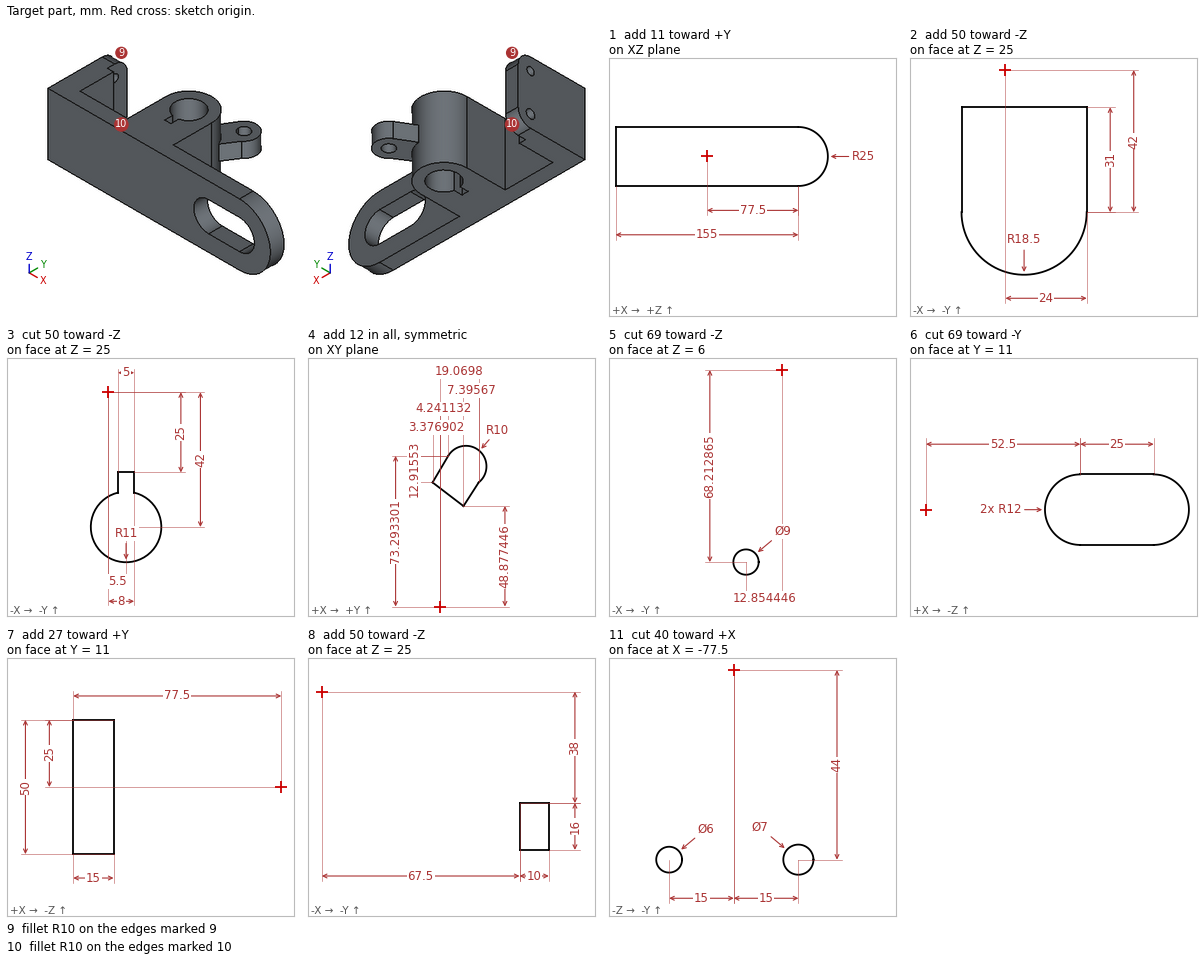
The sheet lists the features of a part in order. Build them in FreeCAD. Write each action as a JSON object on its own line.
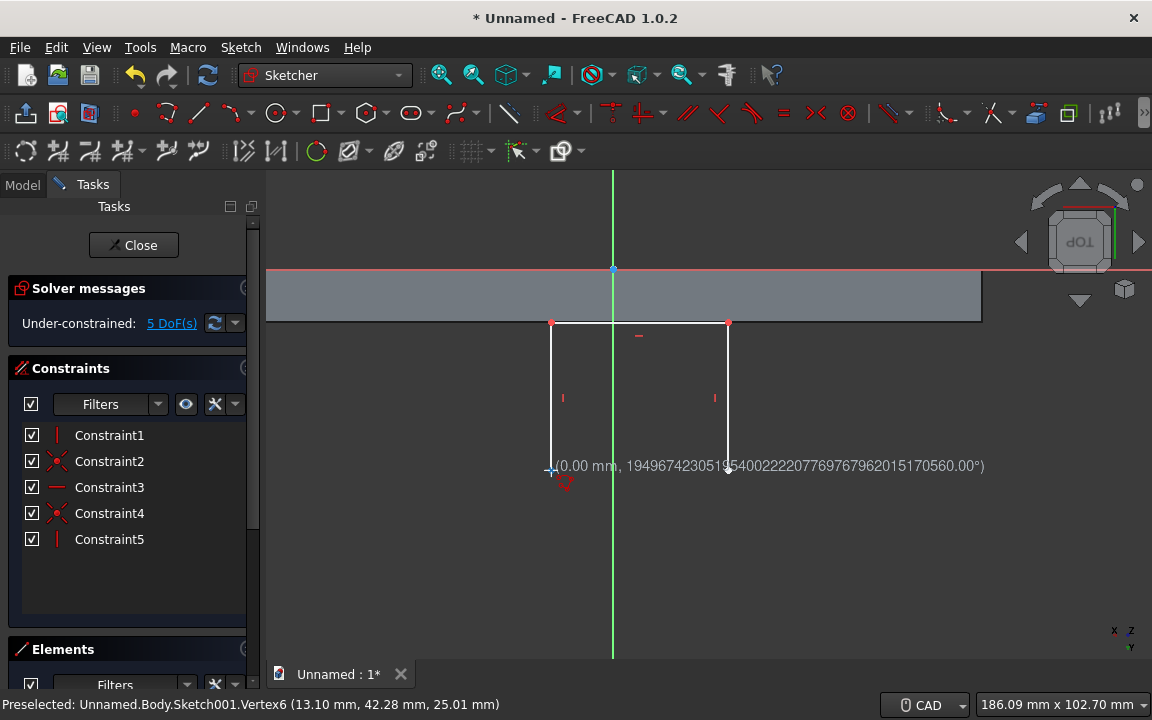
{"action": "left_click", "coordinate": [232, 114]}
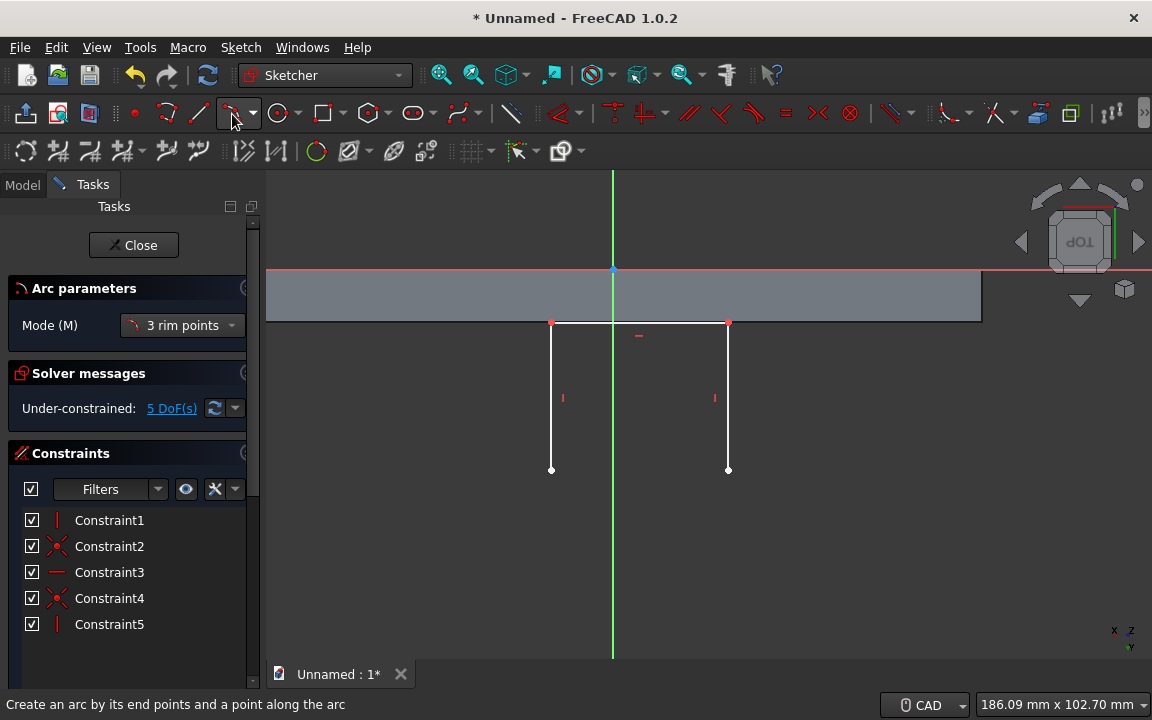
{"action": "left_click", "coordinate": [551, 471]}
{"action": "left_click", "coordinate": [728, 471]}
{"action": "left_click", "coordinate": [640, 558]}
{"action": "key", "text": "Escape"}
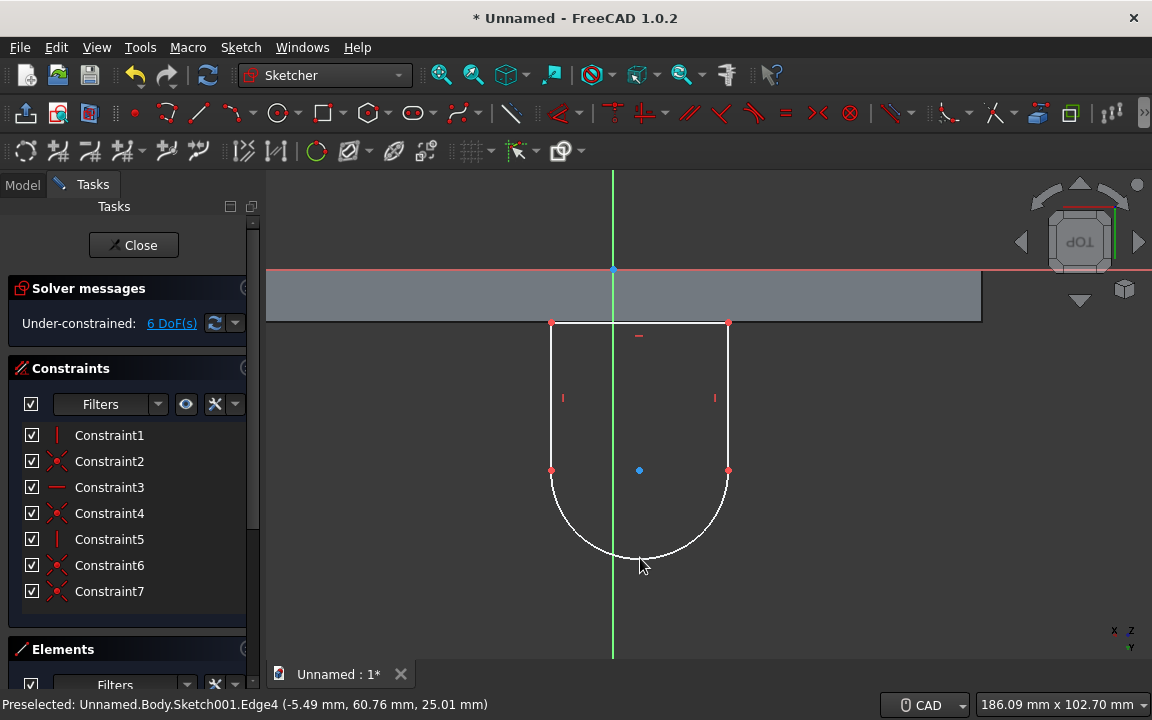
{"action": "left_click", "coordinate": [728, 427]}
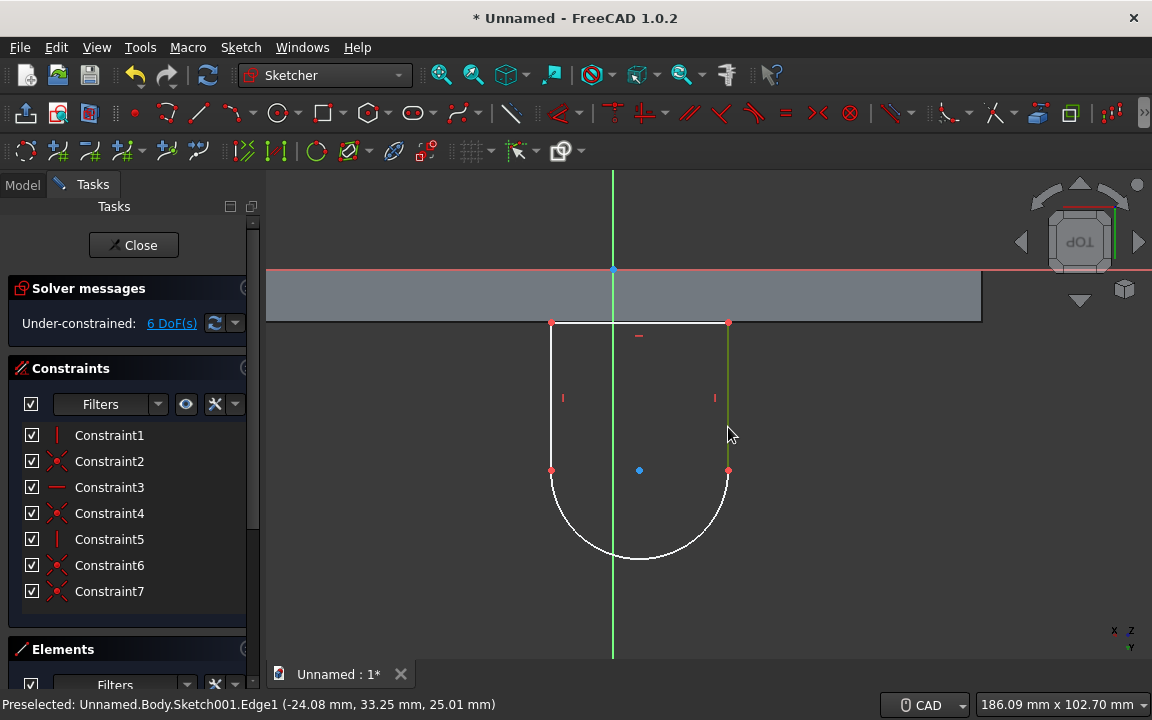
{"action": "left_click", "coordinate": [588, 542]}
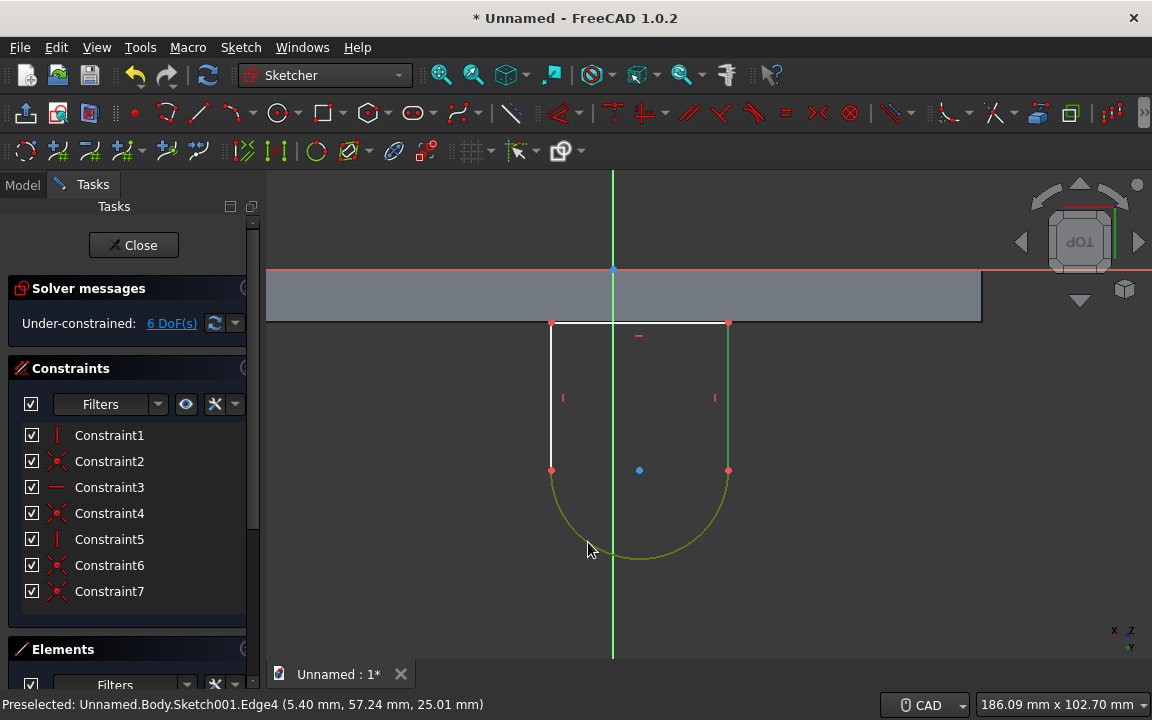
{"action": "left_click", "coordinate": [754, 114]}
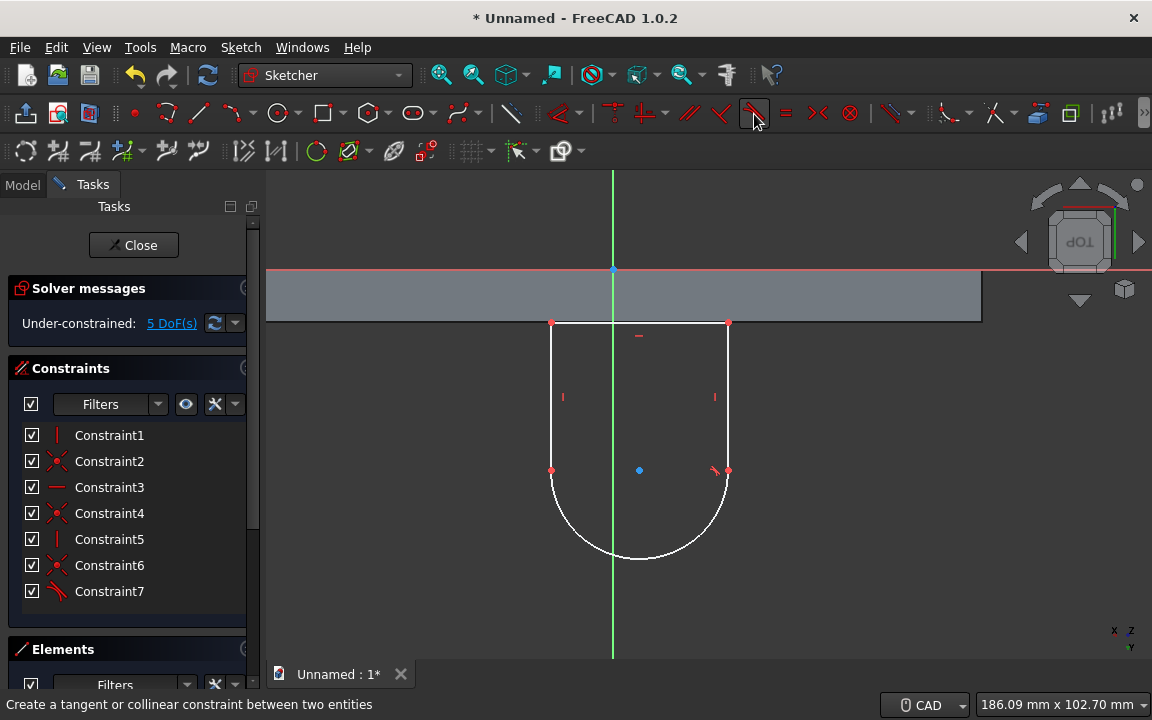
{"action": "left_click", "coordinate": [551, 367]}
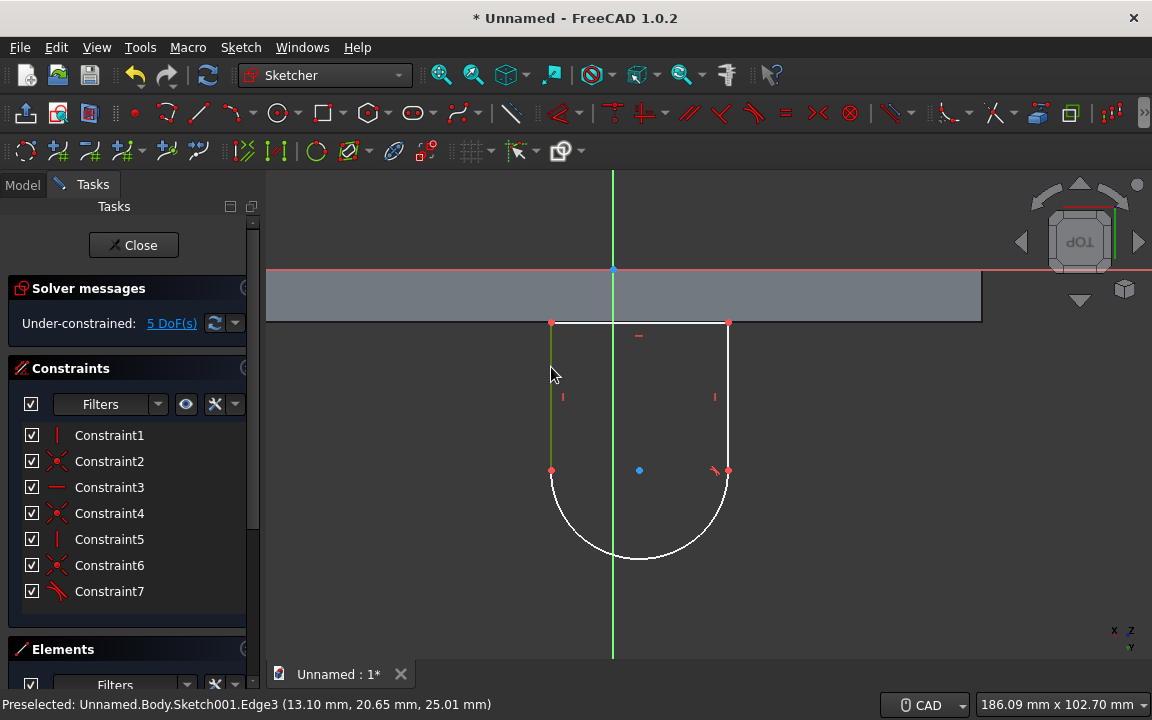
{"action": "left_click", "coordinate": [588, 542]}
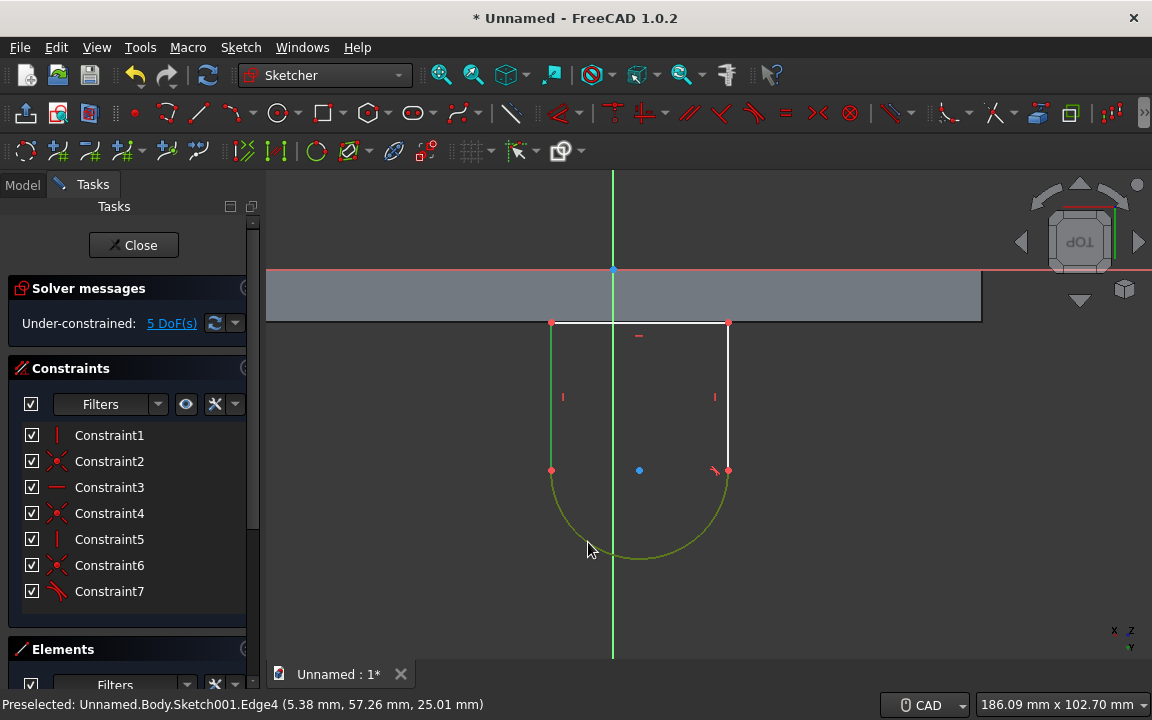
{"action": "left_click", "coordinate": [754, 114]}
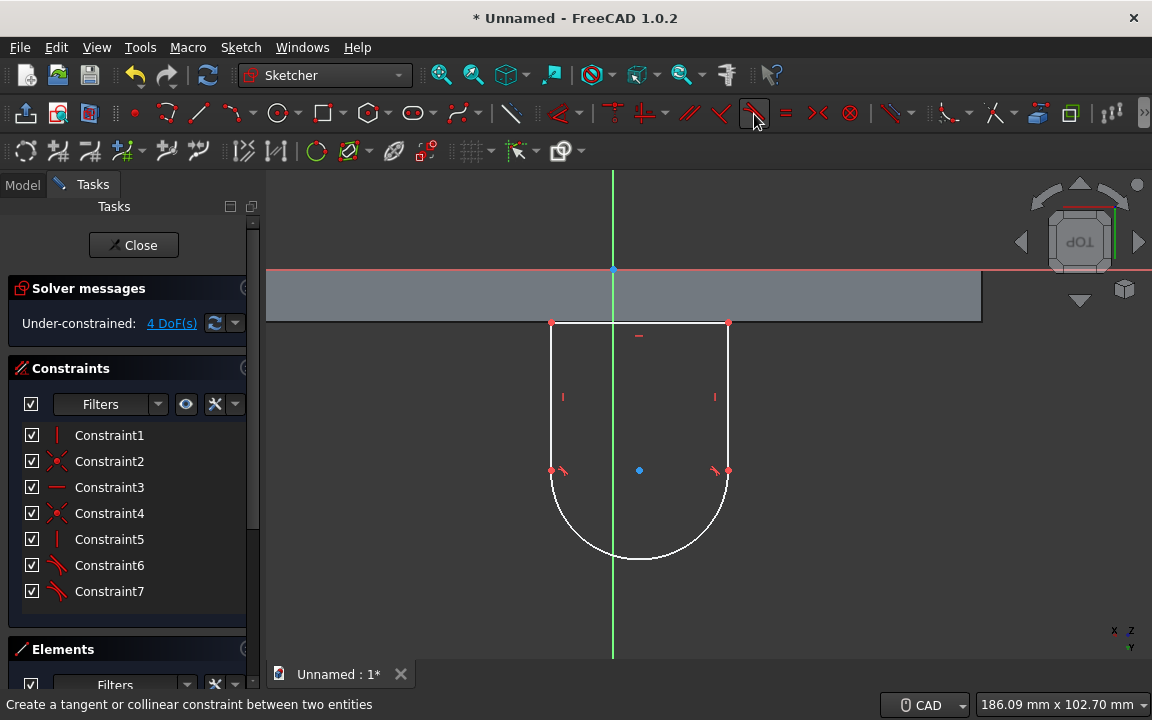
{"action": "left_click", "coordinate": [558, 114]}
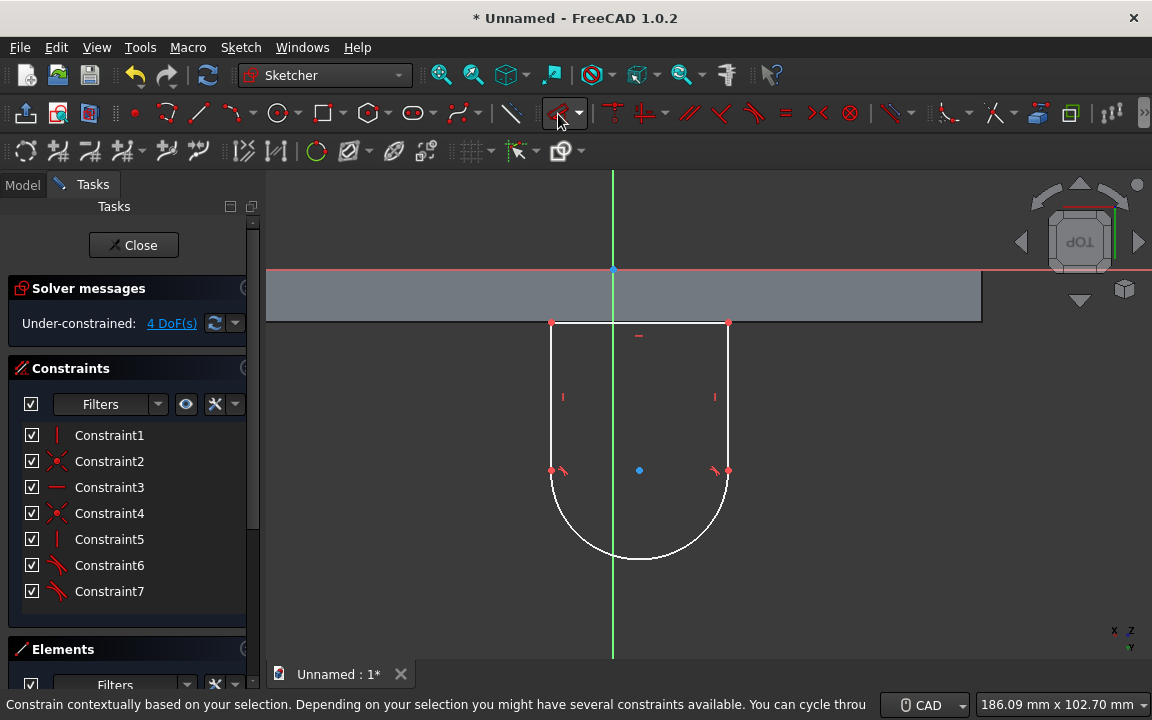
{"action": "left_click", "coordinate": [587, 543]}
{"action": "left_click", "coordinate": [568, 569]}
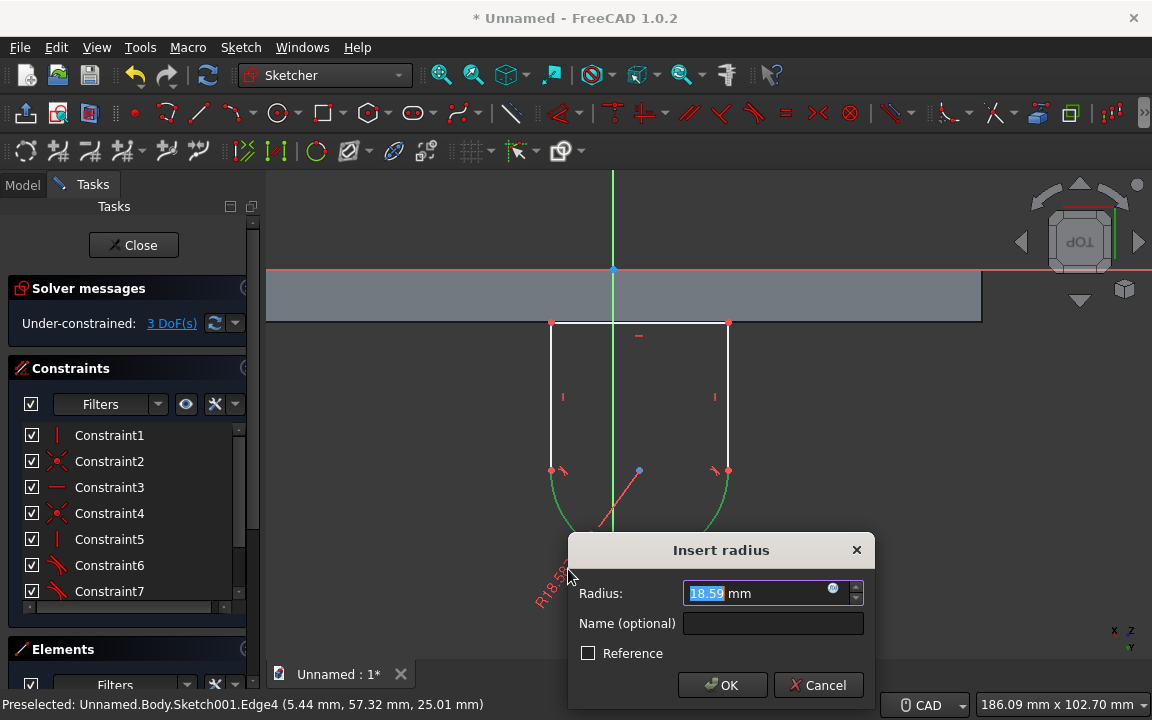
{"action": "type", "text": "18.5"}
{"action": "key", "text": "Return"}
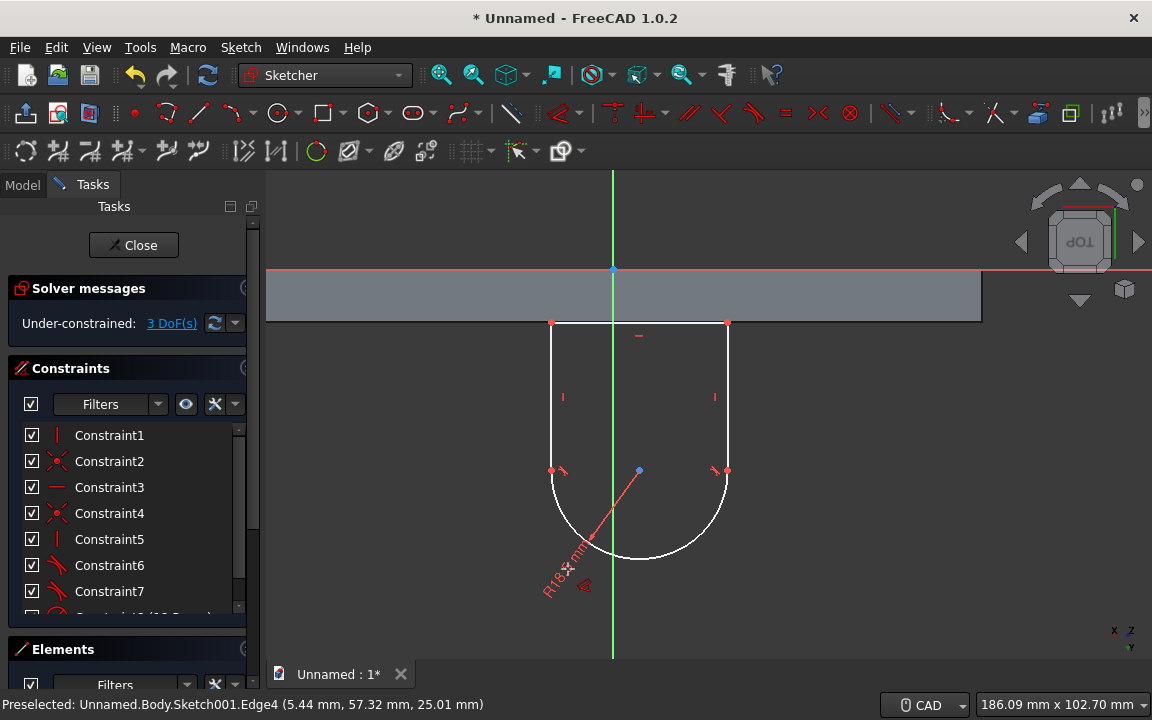
{"action": "left_click", "coordinate": [728, 427]}
{"action": "left_click", "coordinate": [762, 397]}